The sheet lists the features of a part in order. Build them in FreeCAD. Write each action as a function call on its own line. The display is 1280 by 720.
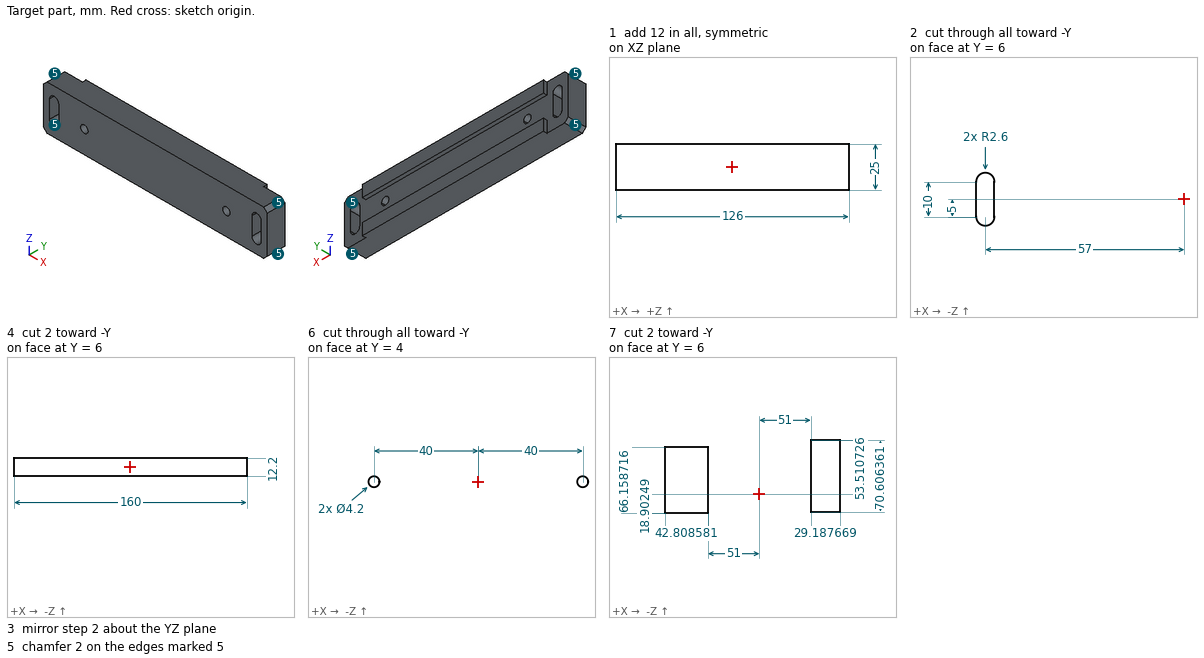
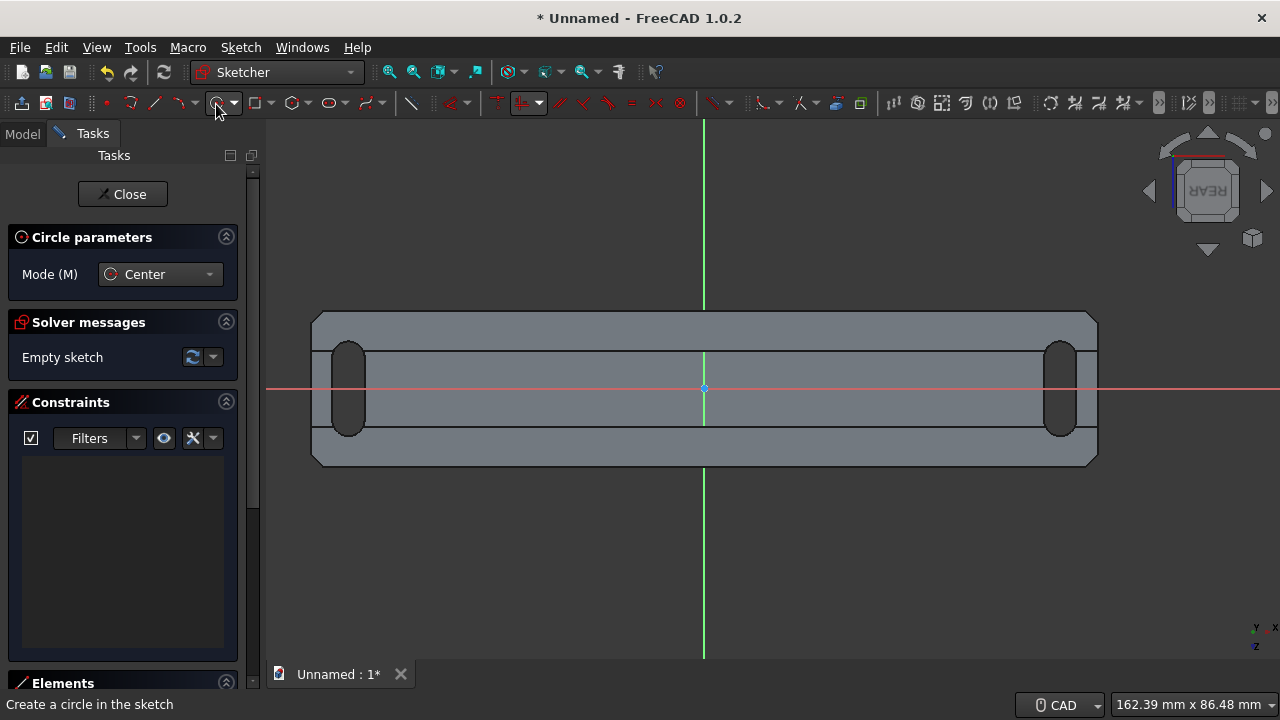
scroll(455, 389, up, 3)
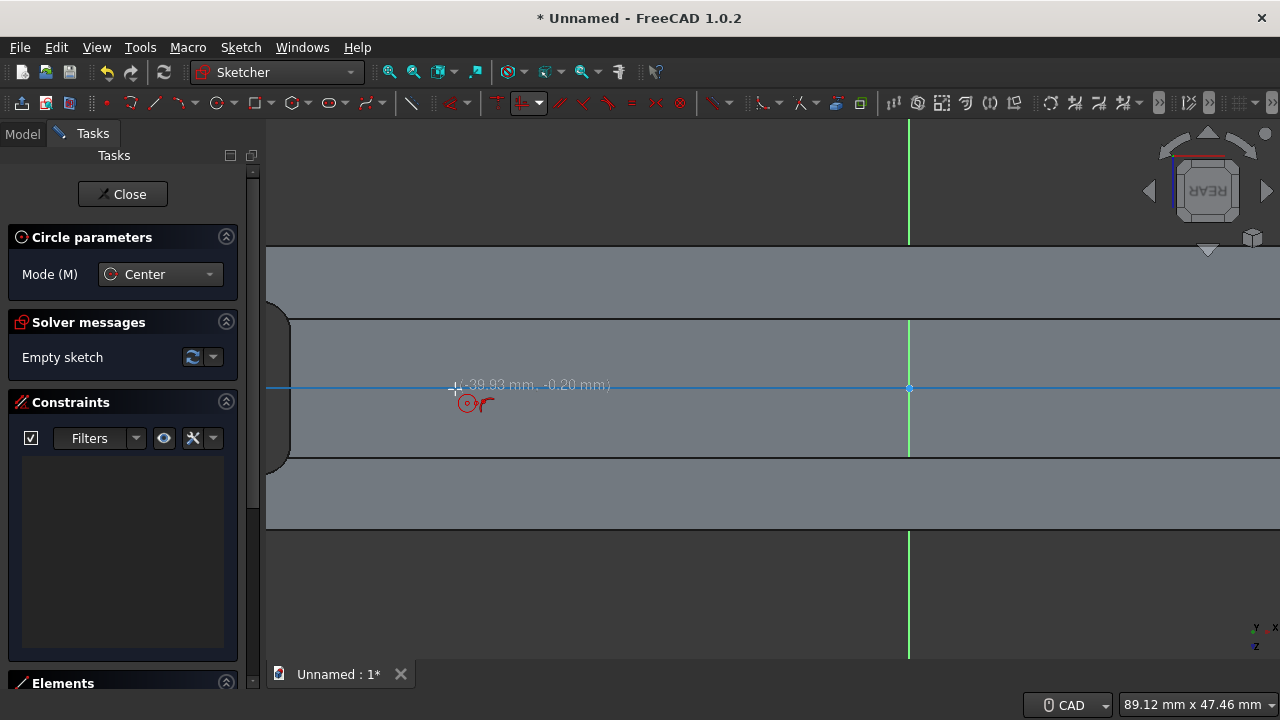
click(454, 388)
click(471, 371)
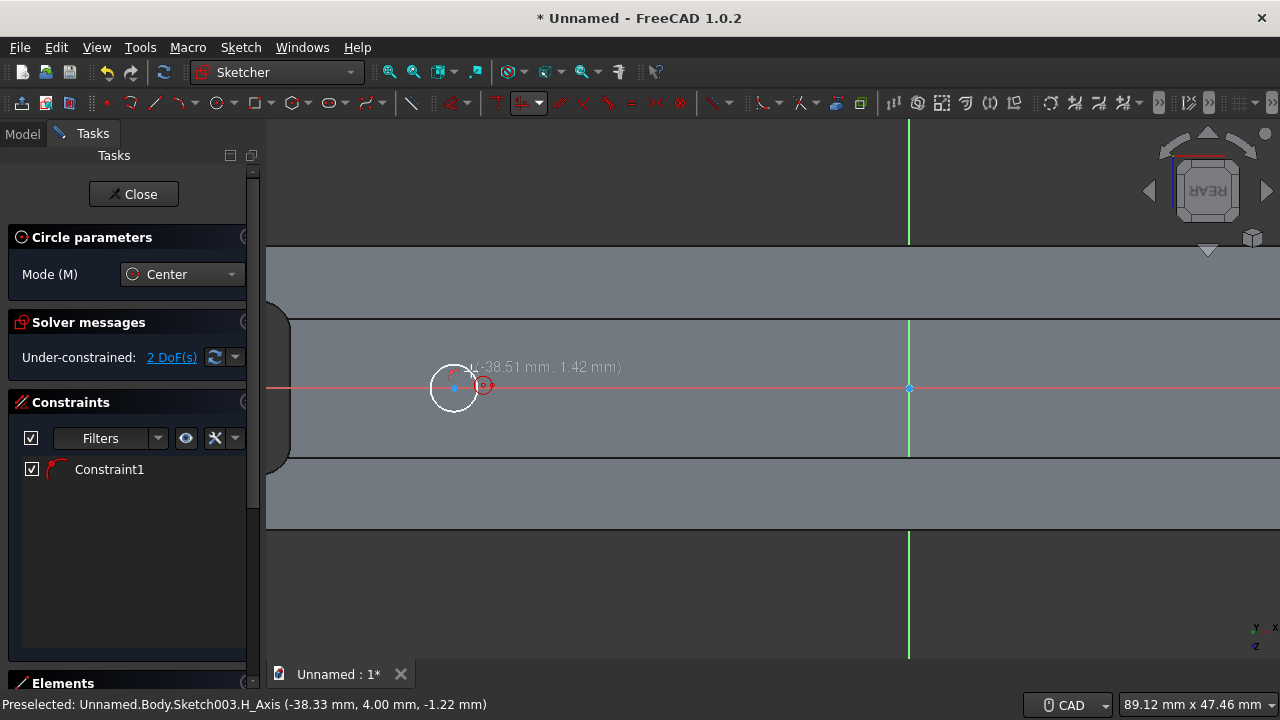
scroll(456, 390, down, 3)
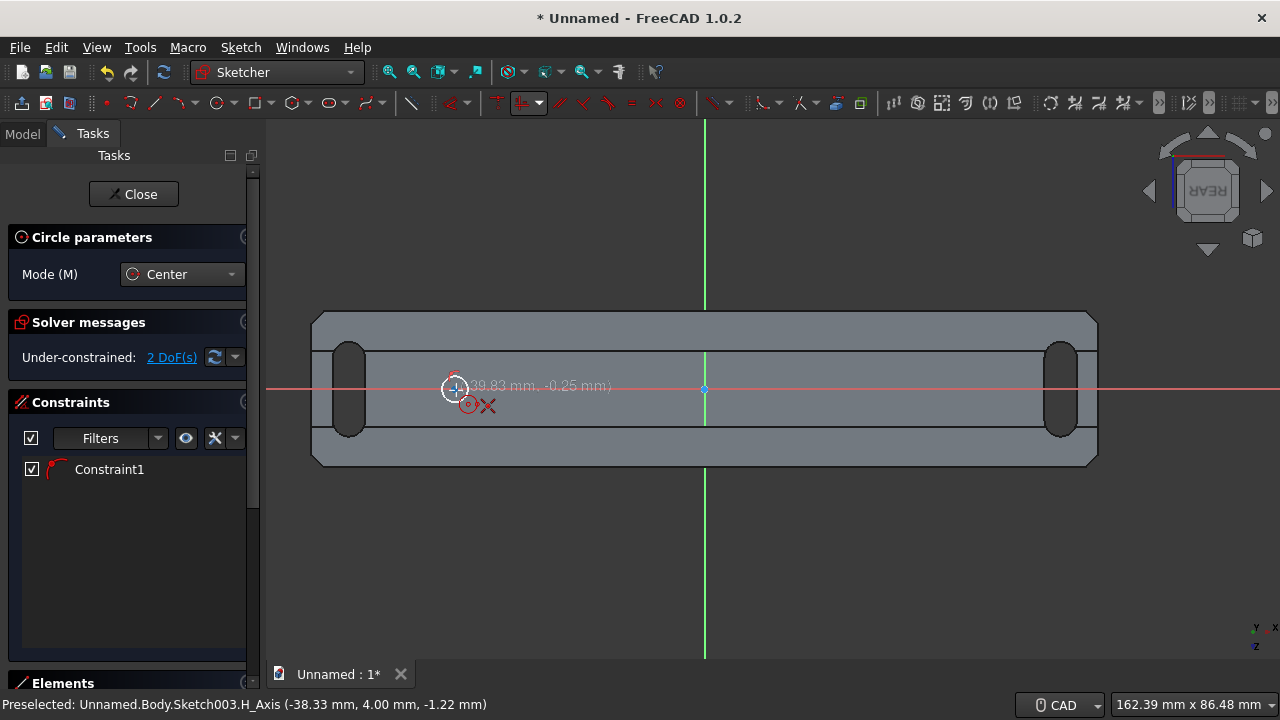
scroll(955, 389, up, 3)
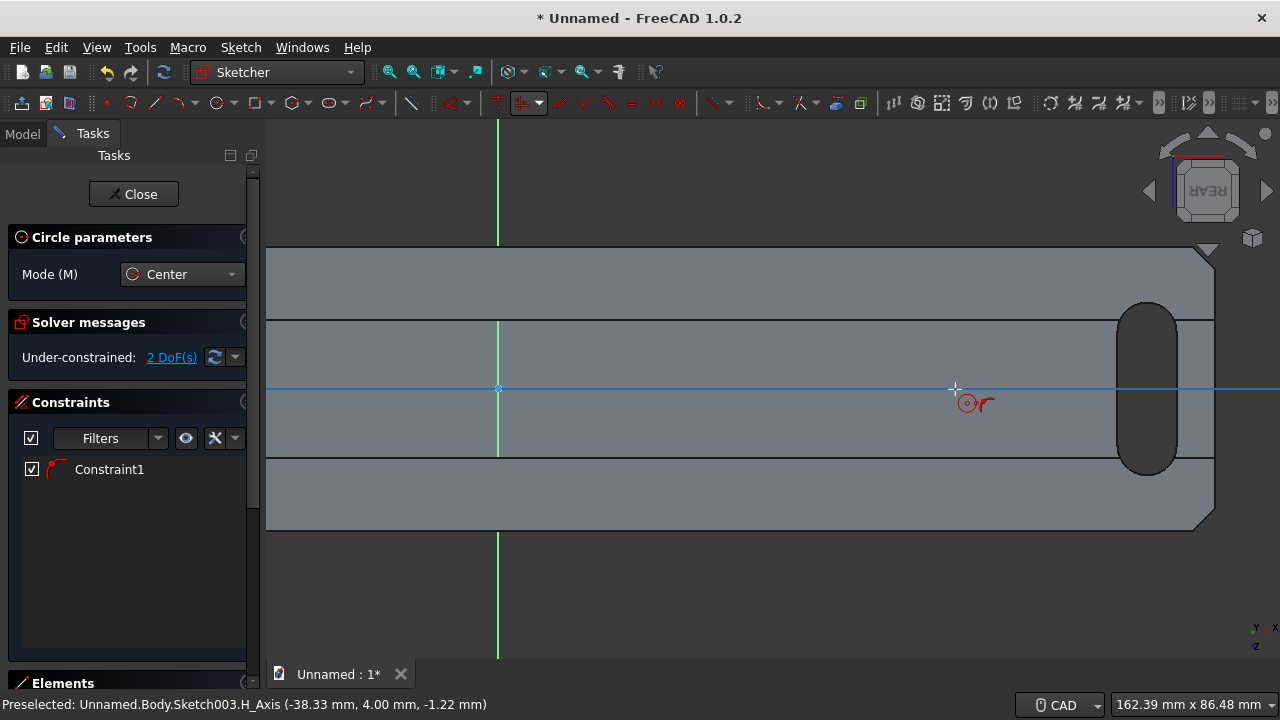
click(954, 389)
click(970, 372)
key(Escape)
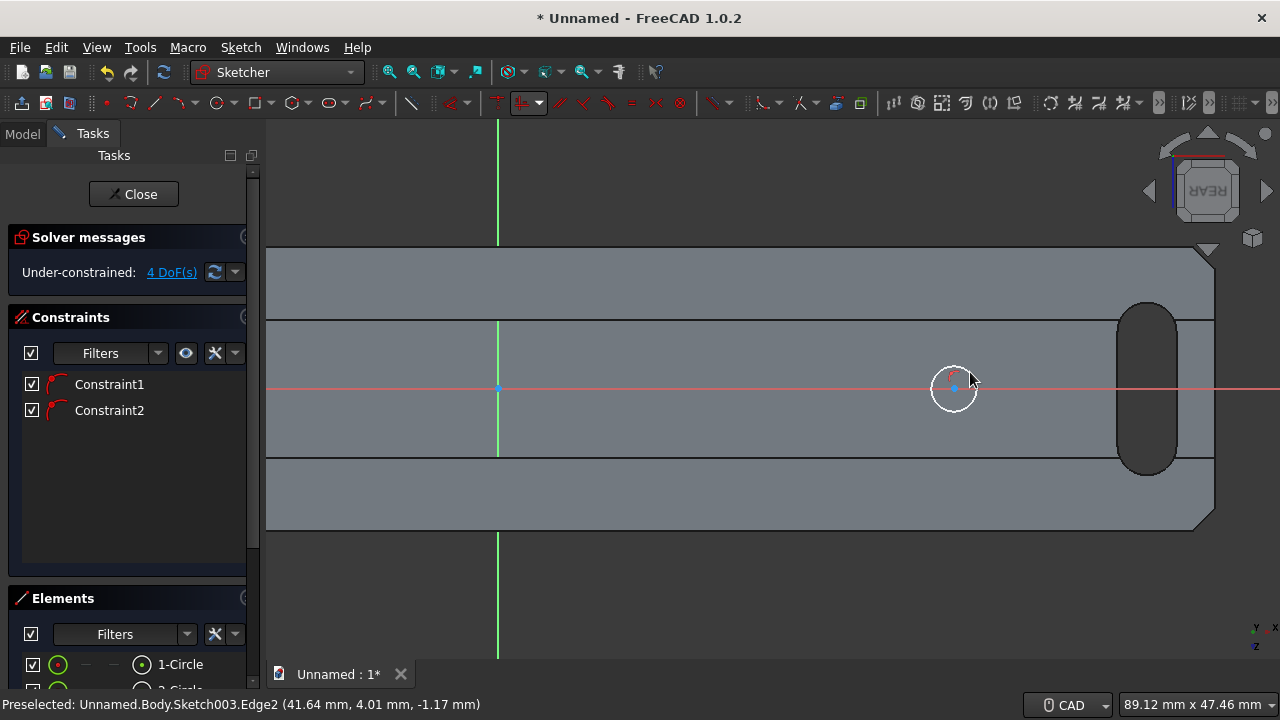
scroll(955, 389, down, 3)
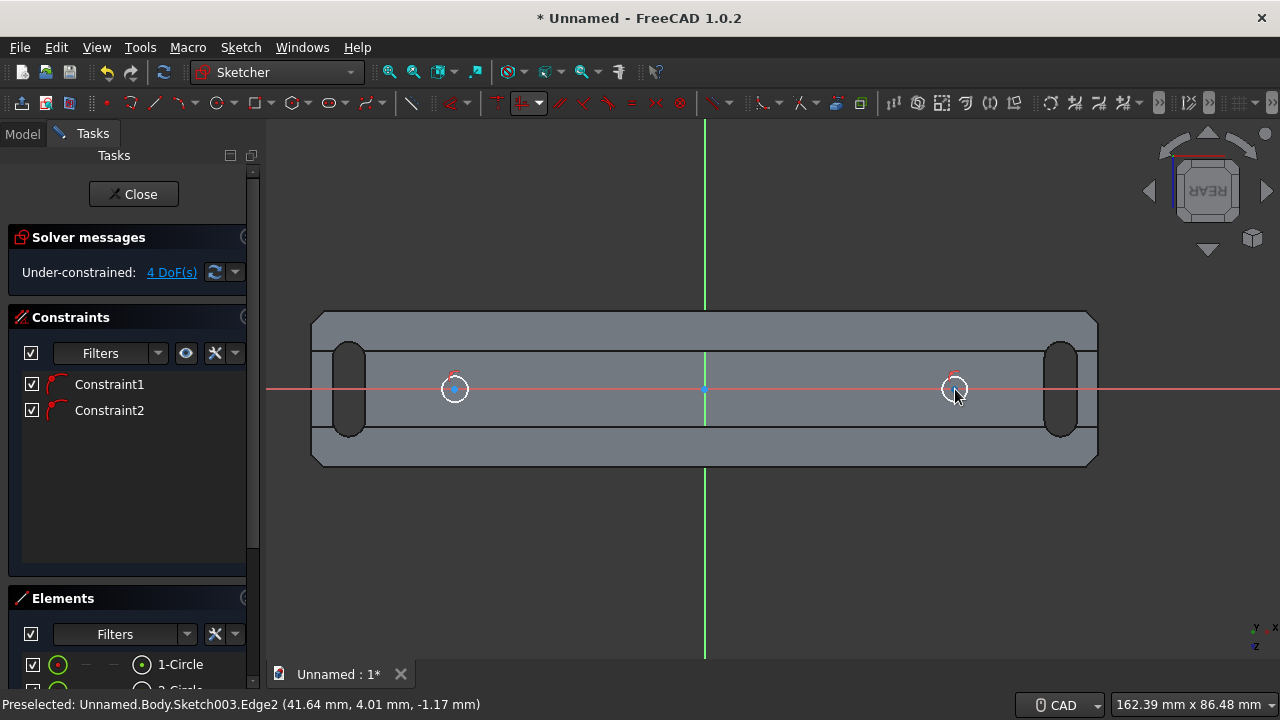
scroll(464, 380, up, 3)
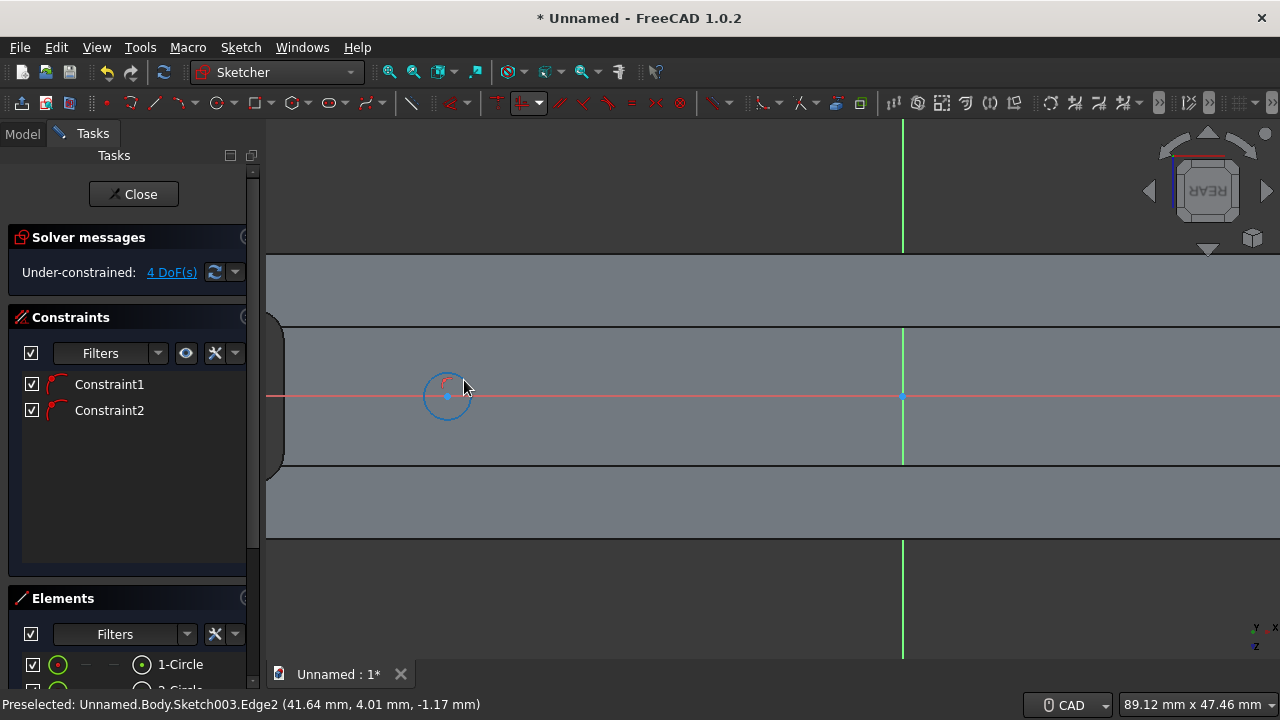
click(464, 380)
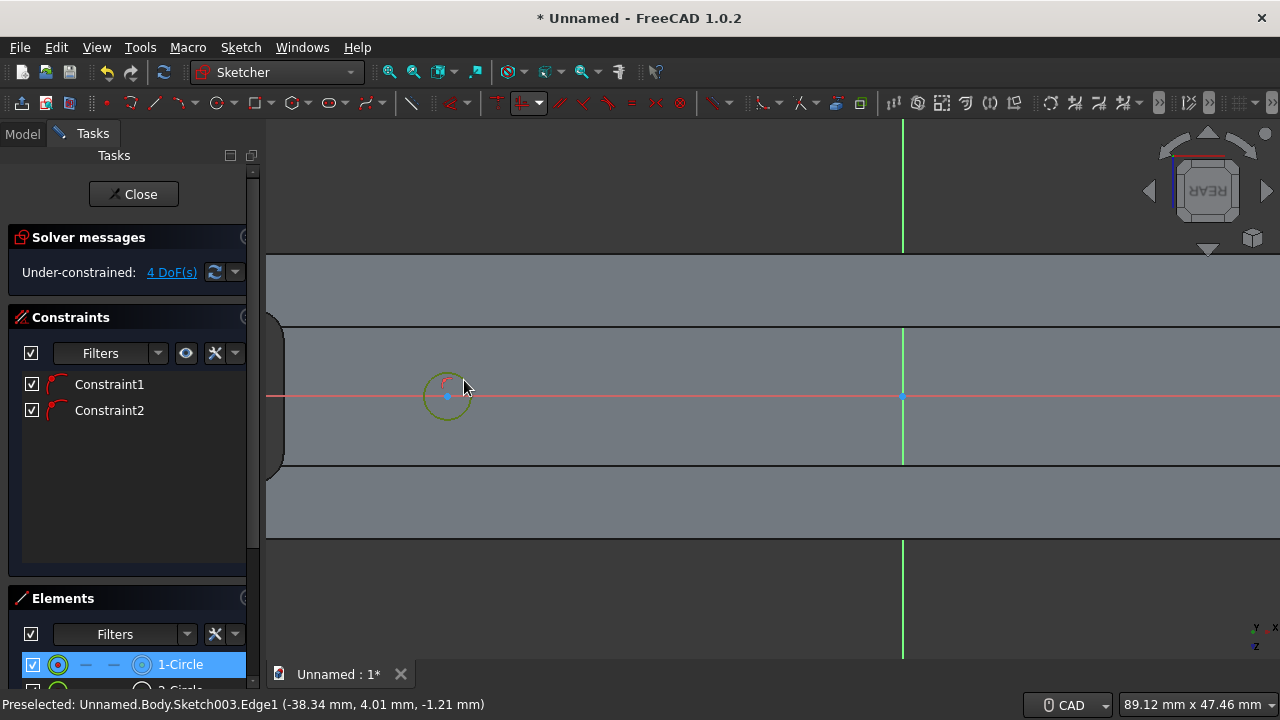
scroll(464, 380, down, 3)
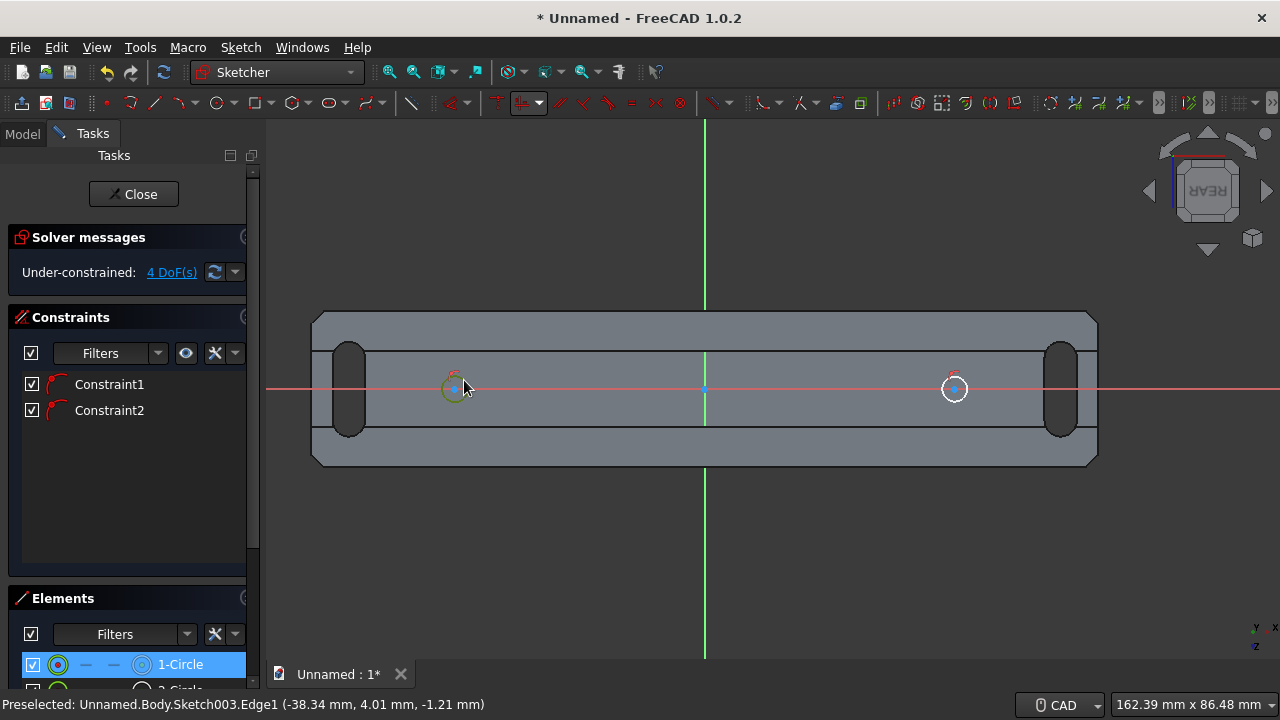
scroll(964, 380, up, 3)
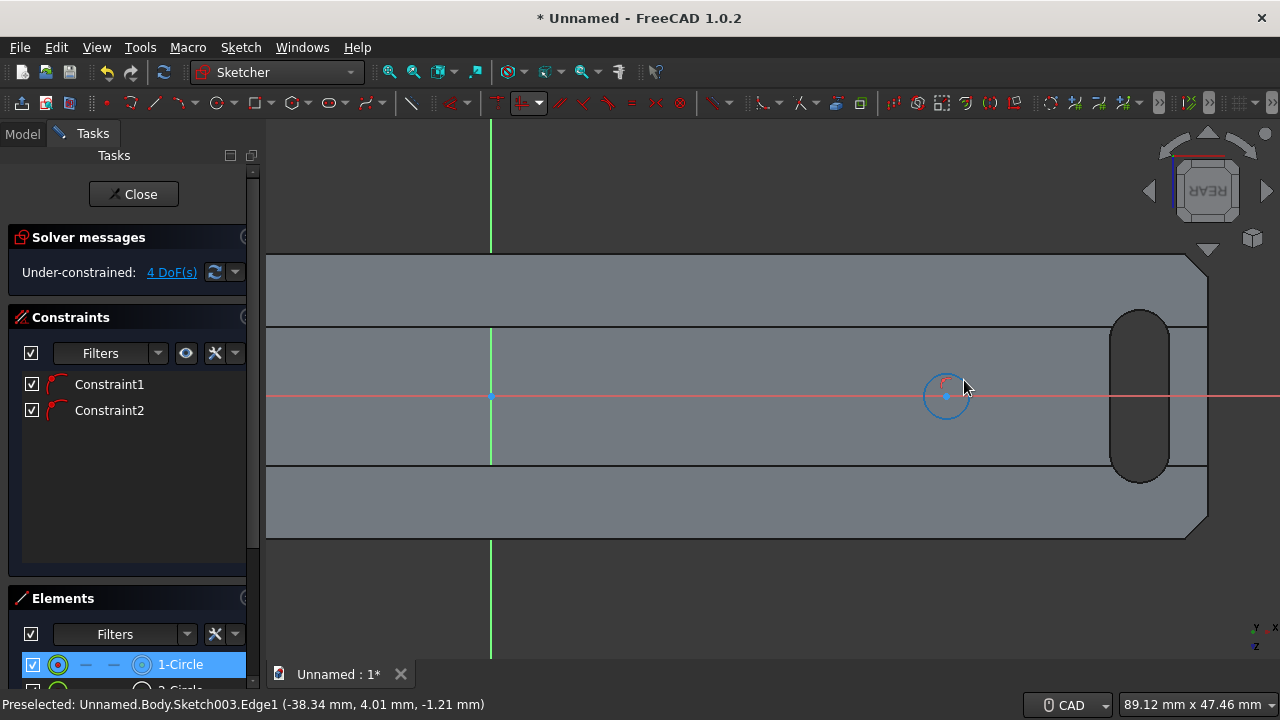
click(963, 380)